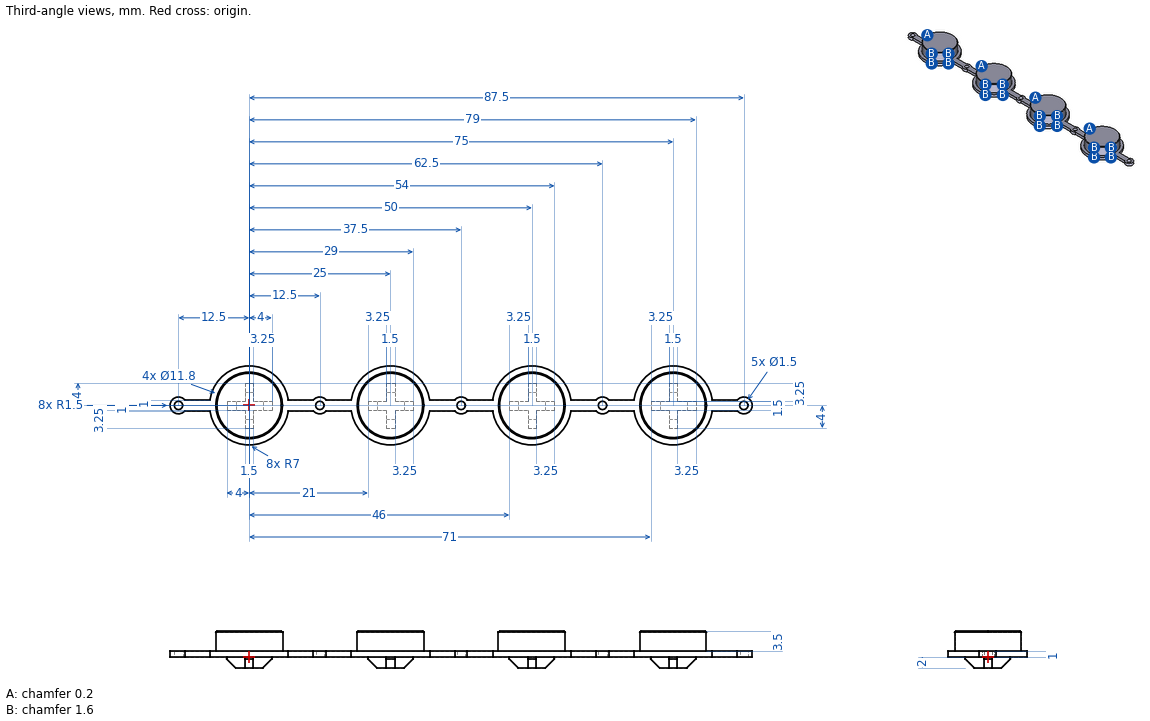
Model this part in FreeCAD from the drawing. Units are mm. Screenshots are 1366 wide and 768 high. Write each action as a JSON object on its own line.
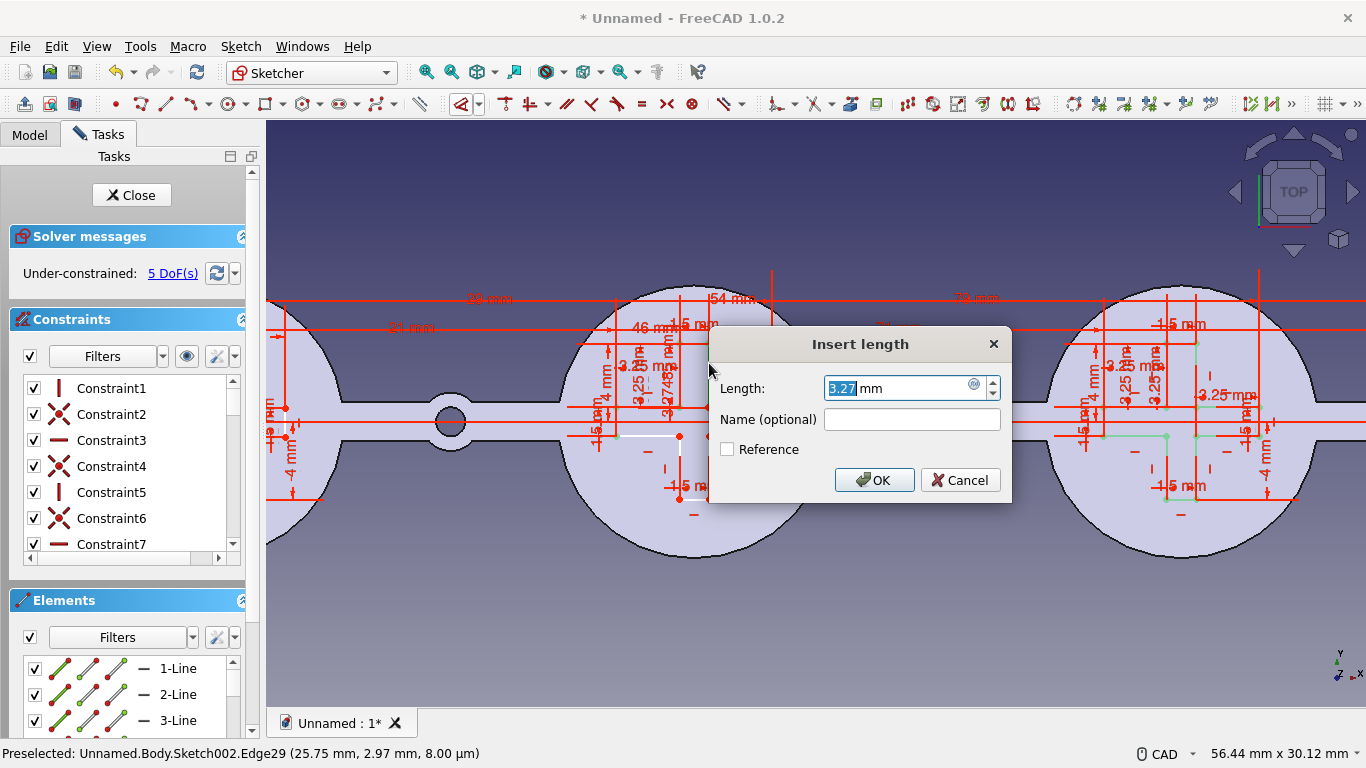
{"action": "type", "text": "3.25"}
{"action": "key", "text": "Return"}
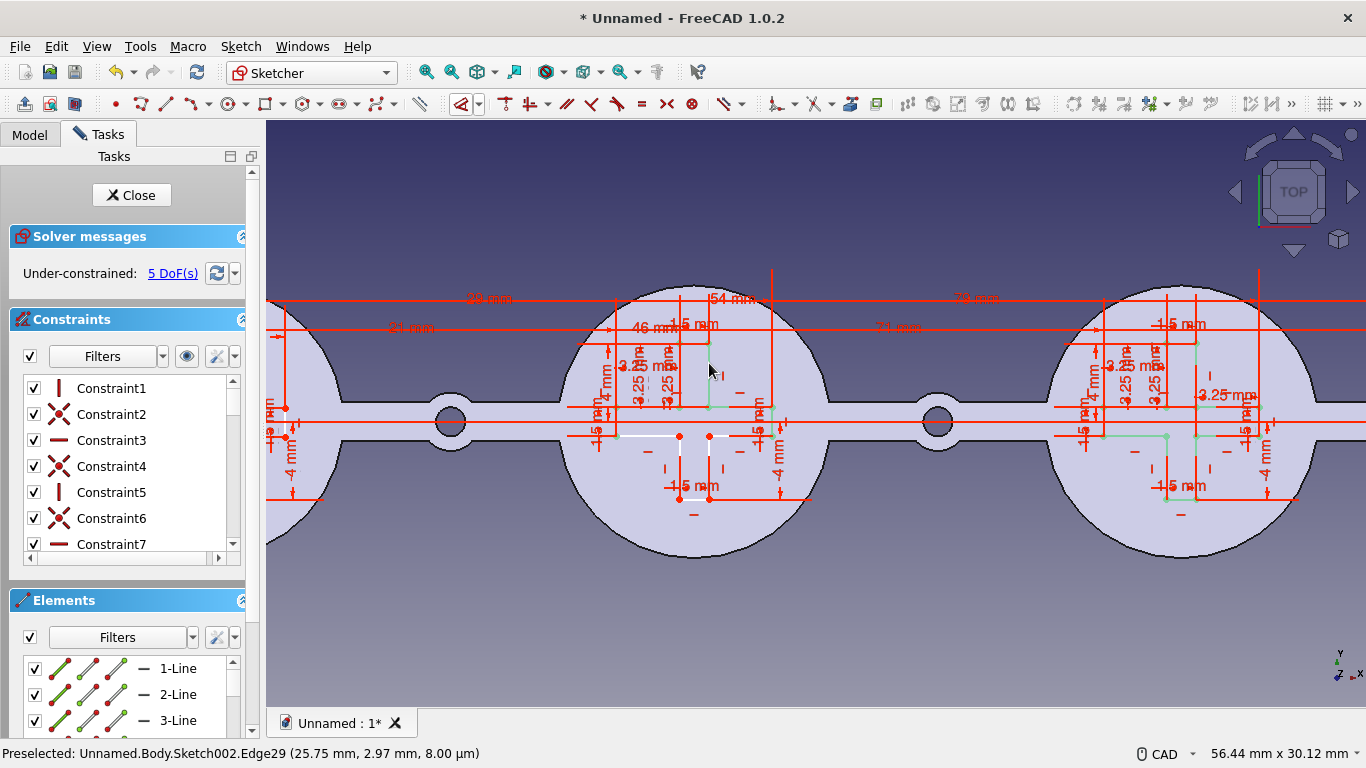
{"action": "left_click", "coordinate": [728, 436]}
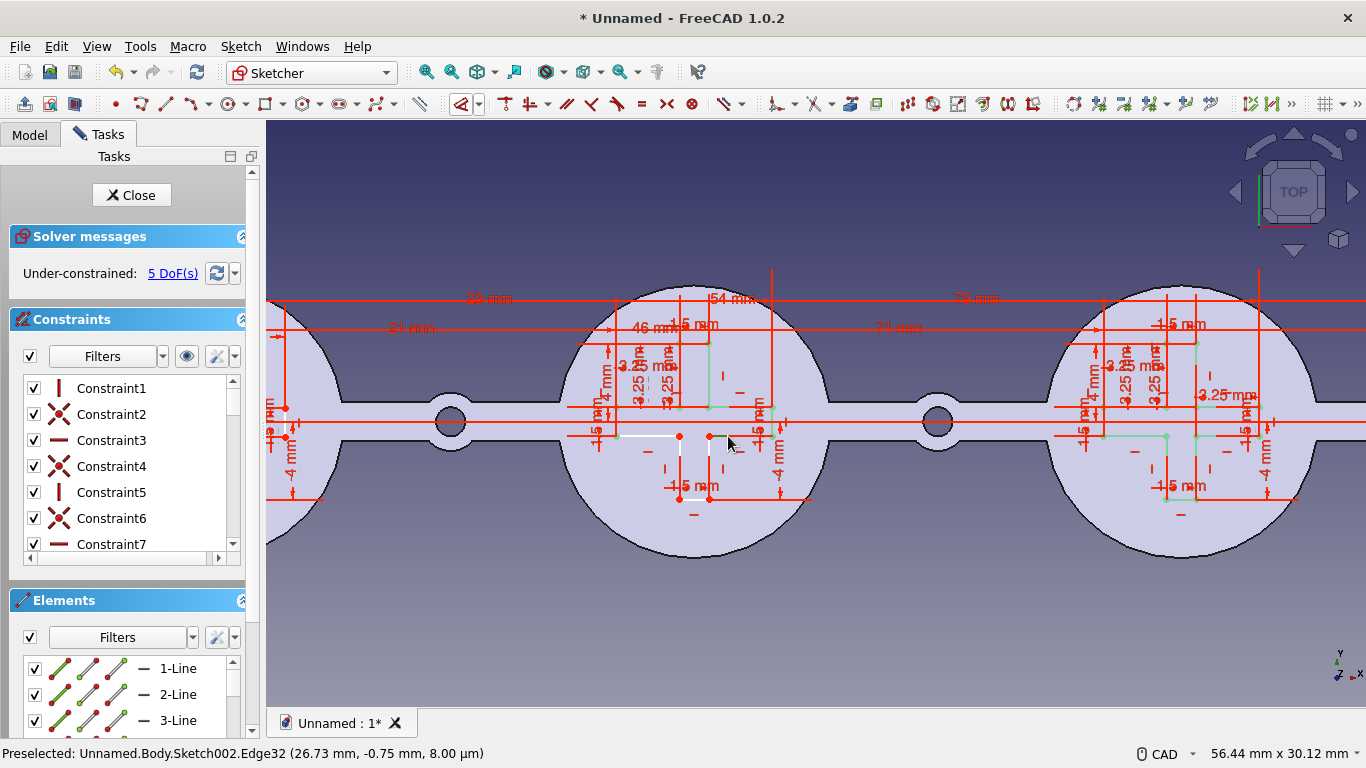
{"action": "key", "text": "l"}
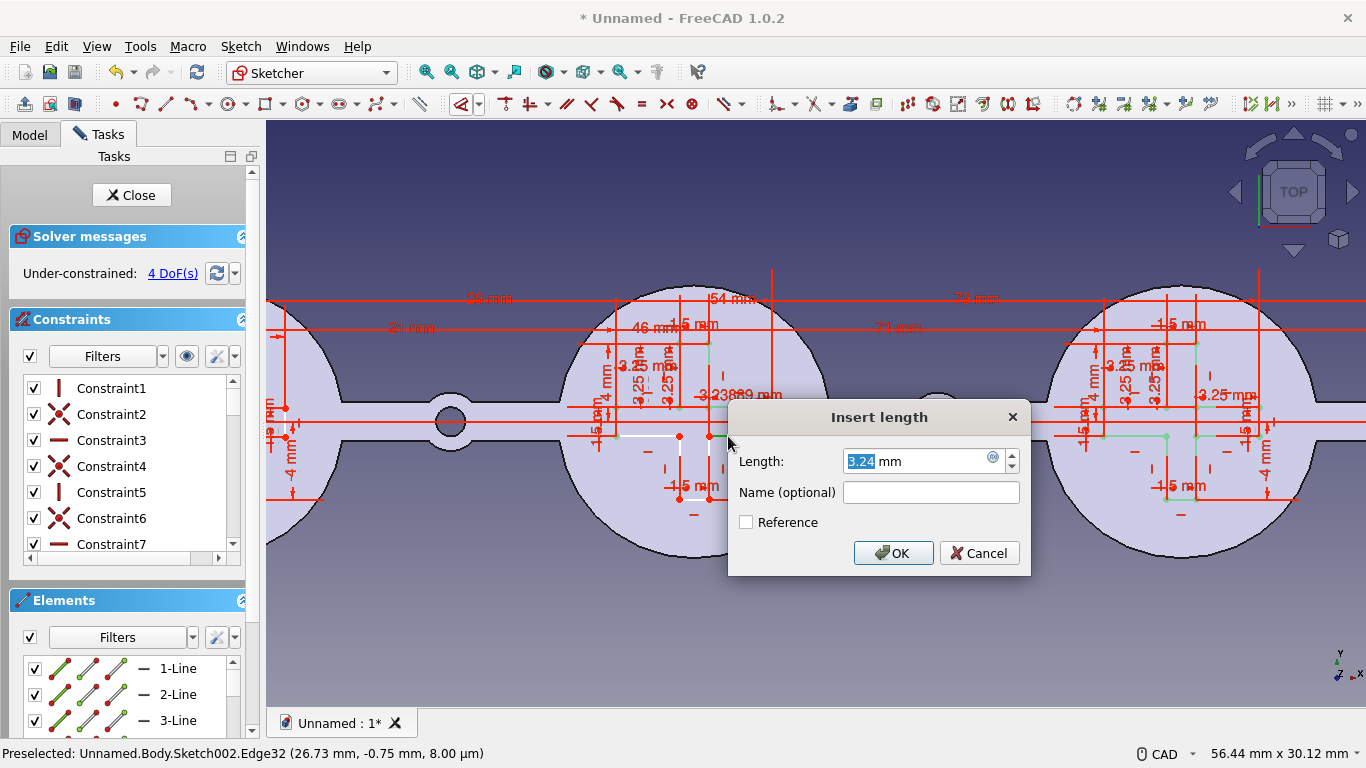
{"action": "type", "text": "3.25"}
{"action": "key", "text": "Return"}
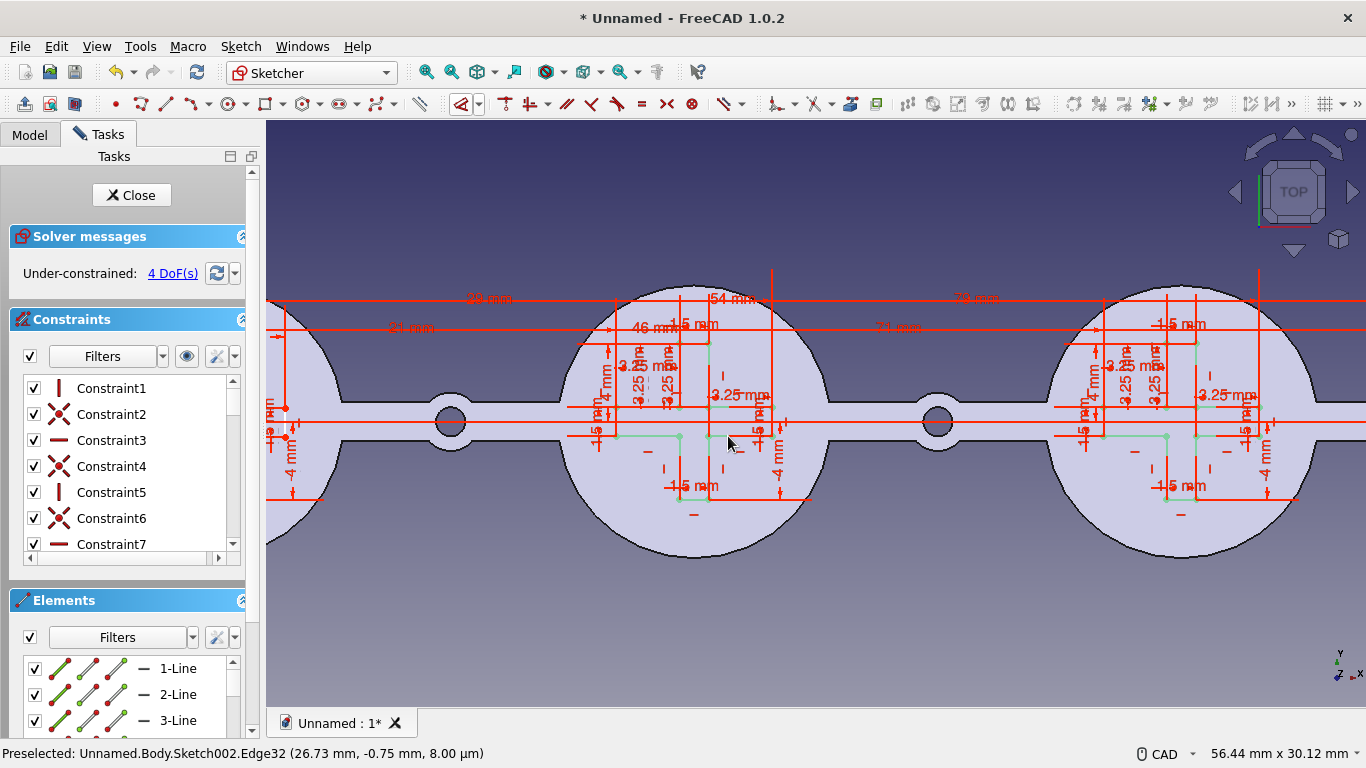
{"action": "scroll", "coordinate": [637, 409], "scroll_direction": "down", "scroll_amount": 5}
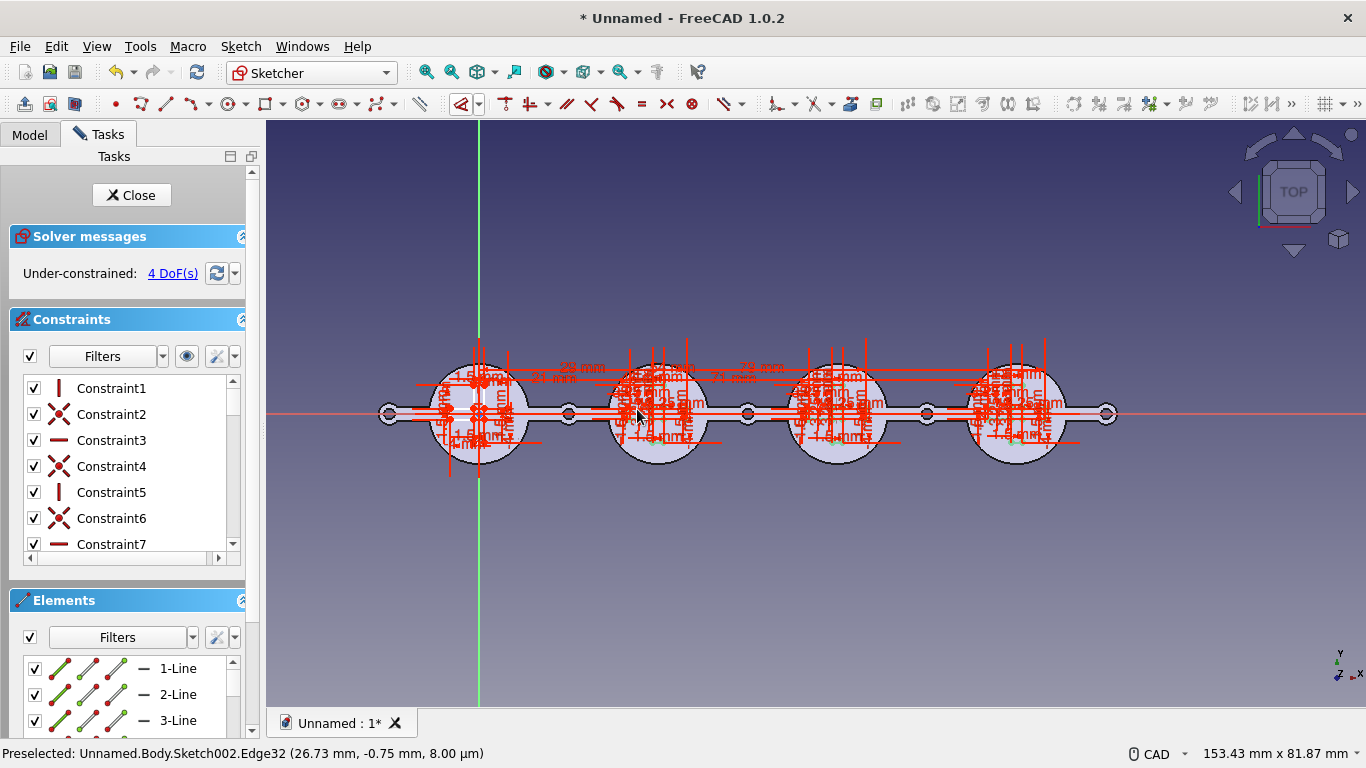
{"action": "scroll", "coordinate": [491, 409], "scroll_direction": "up", "scroll_amount": 6}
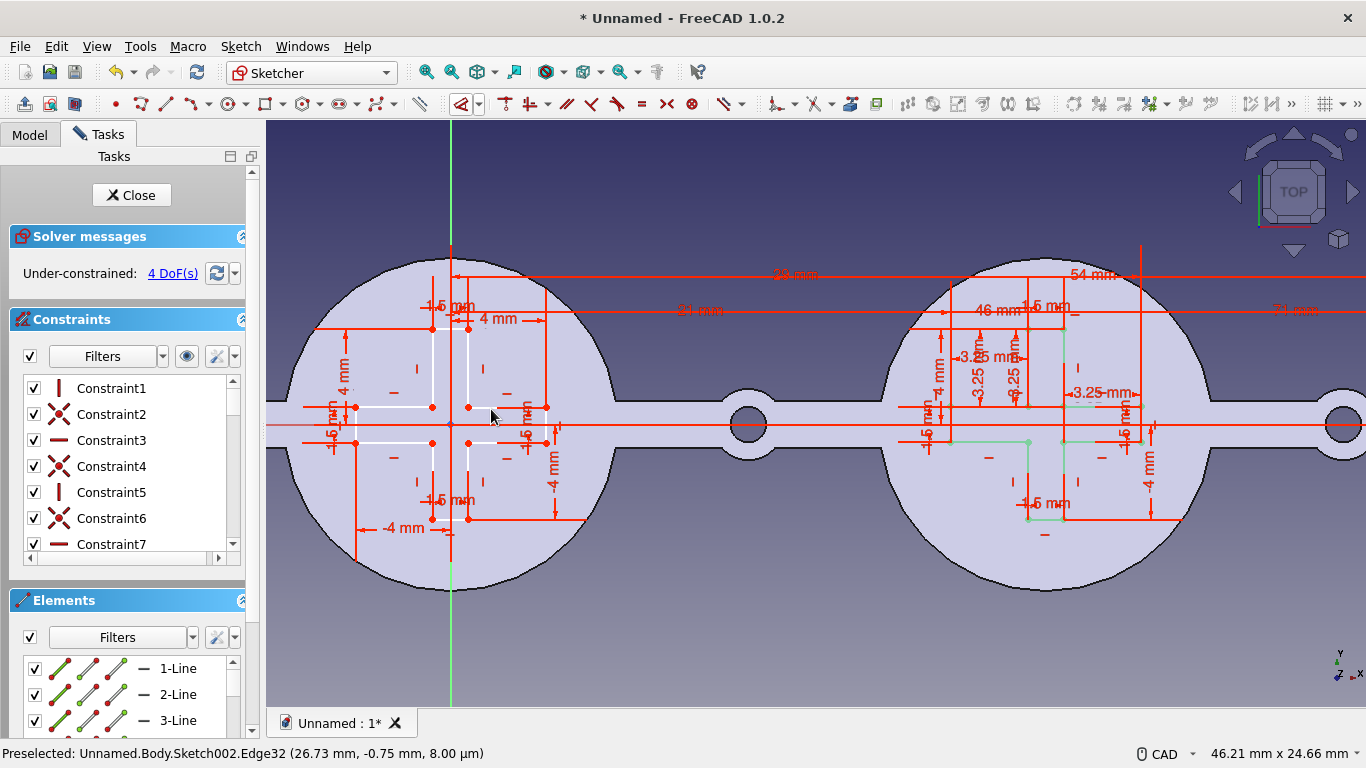
{"action": "left_click", "coordinate": [492, 408]}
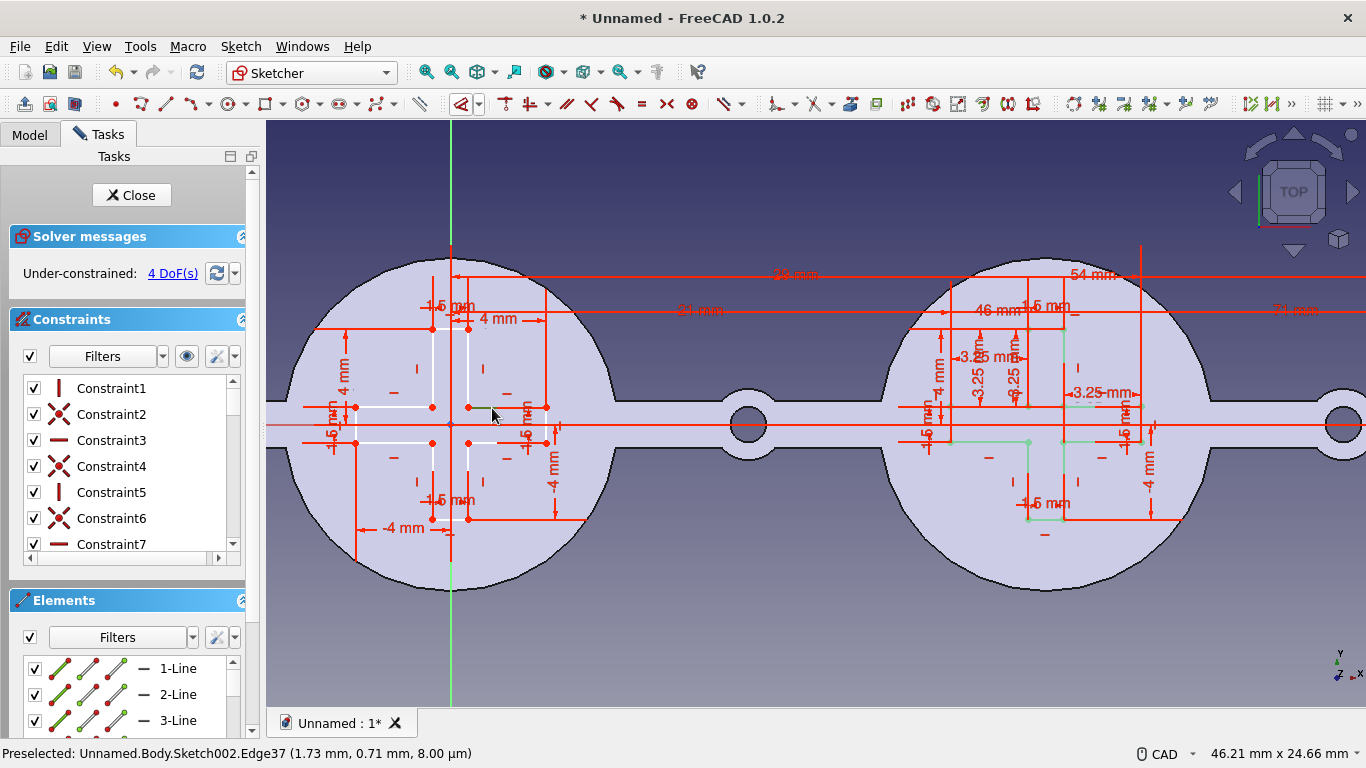
{"action": "key", "text": "l"}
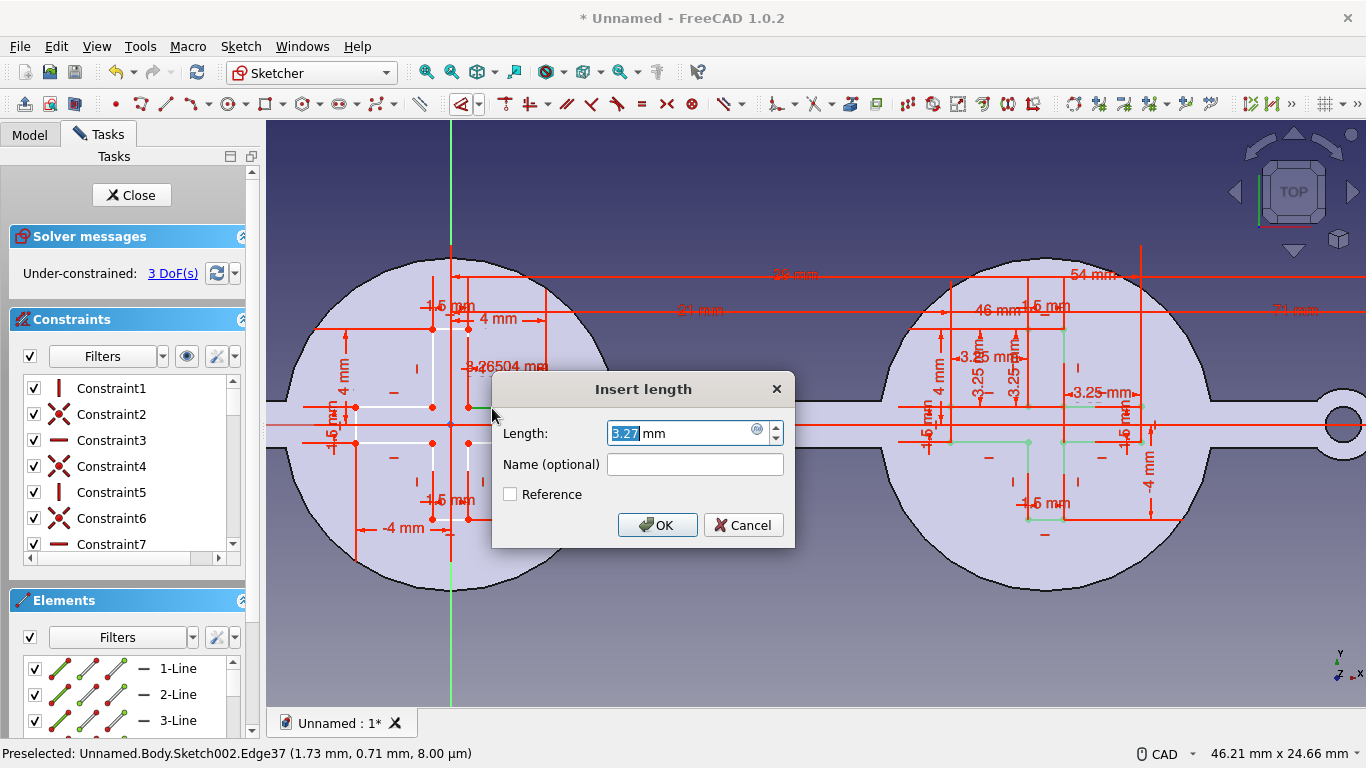
{"action": "type", "text": "3.25"}
{"action": "key", "text": "Return"}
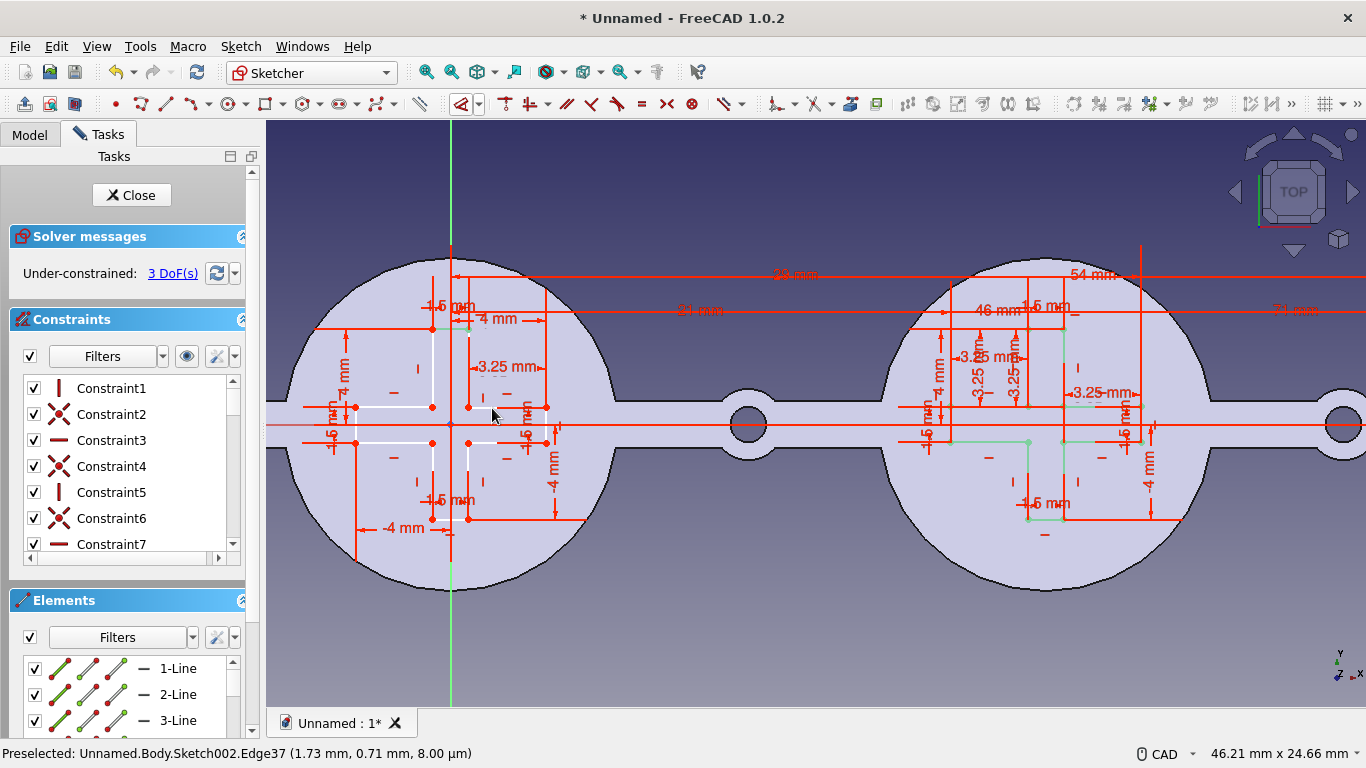
{"action": "left_click", "coordinate": [492, 443]}